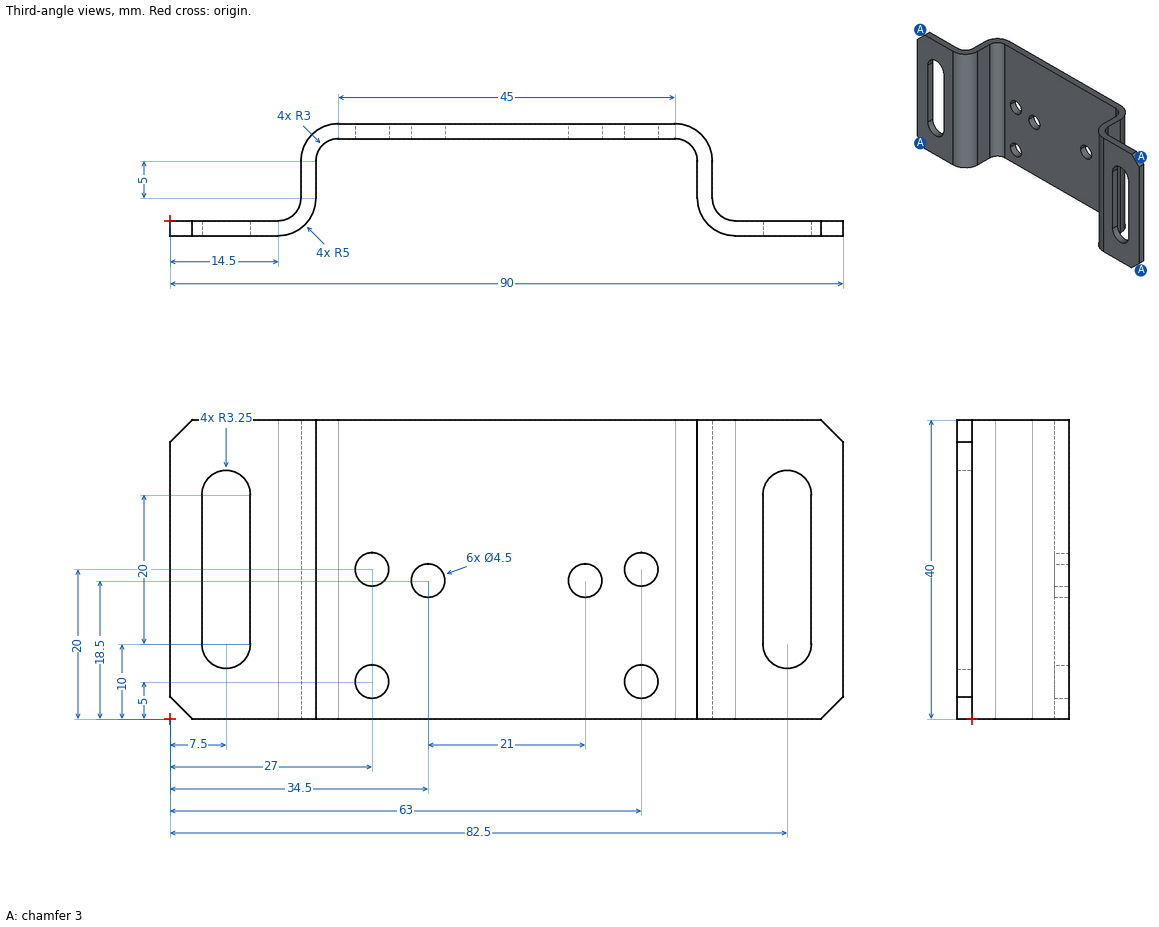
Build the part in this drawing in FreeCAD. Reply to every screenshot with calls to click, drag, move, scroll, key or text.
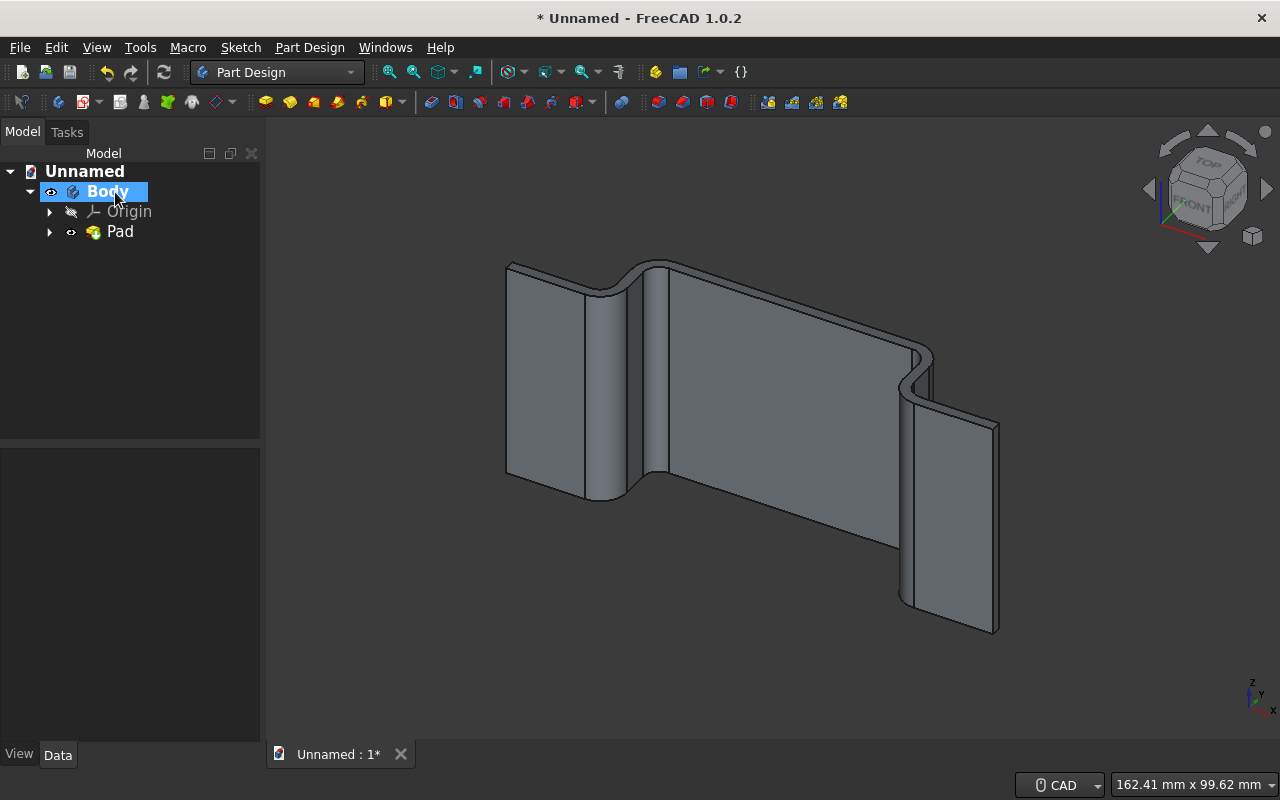
click(998, 424)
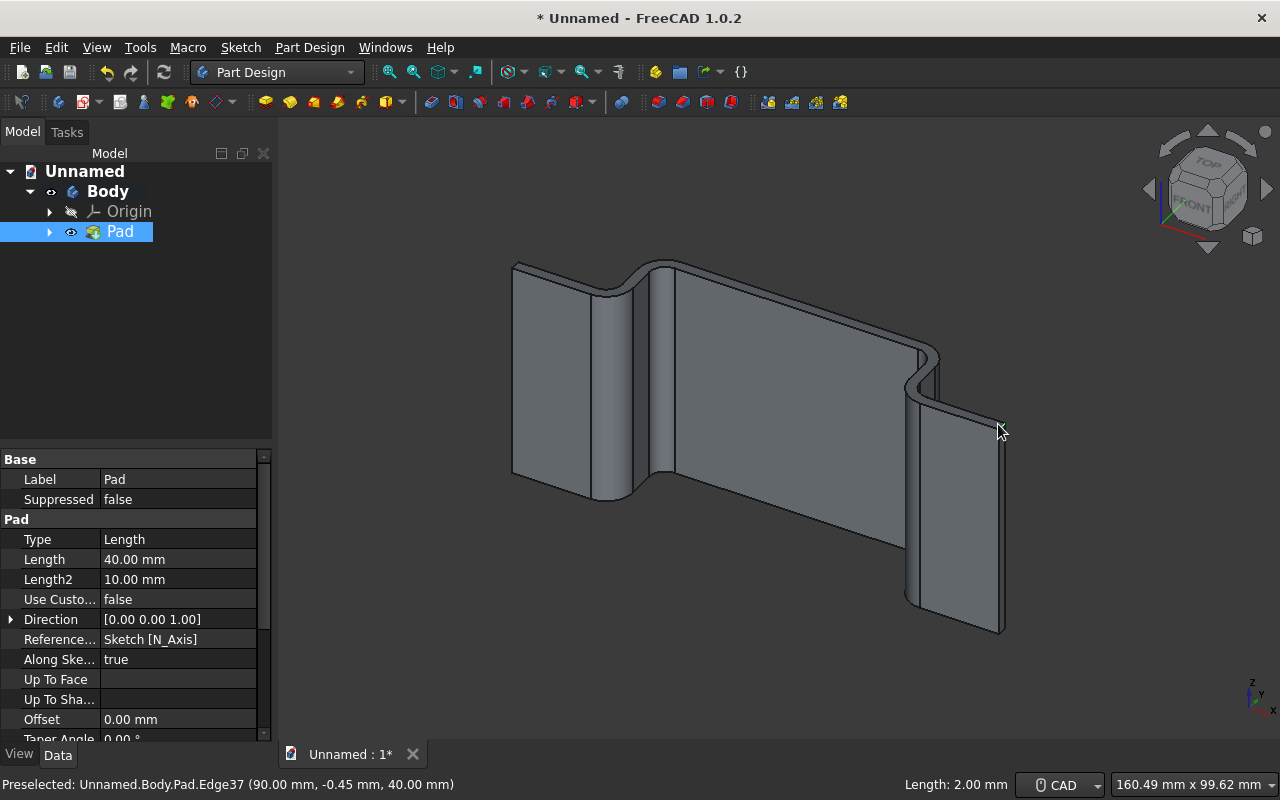
scroll(515, 469, up, 6)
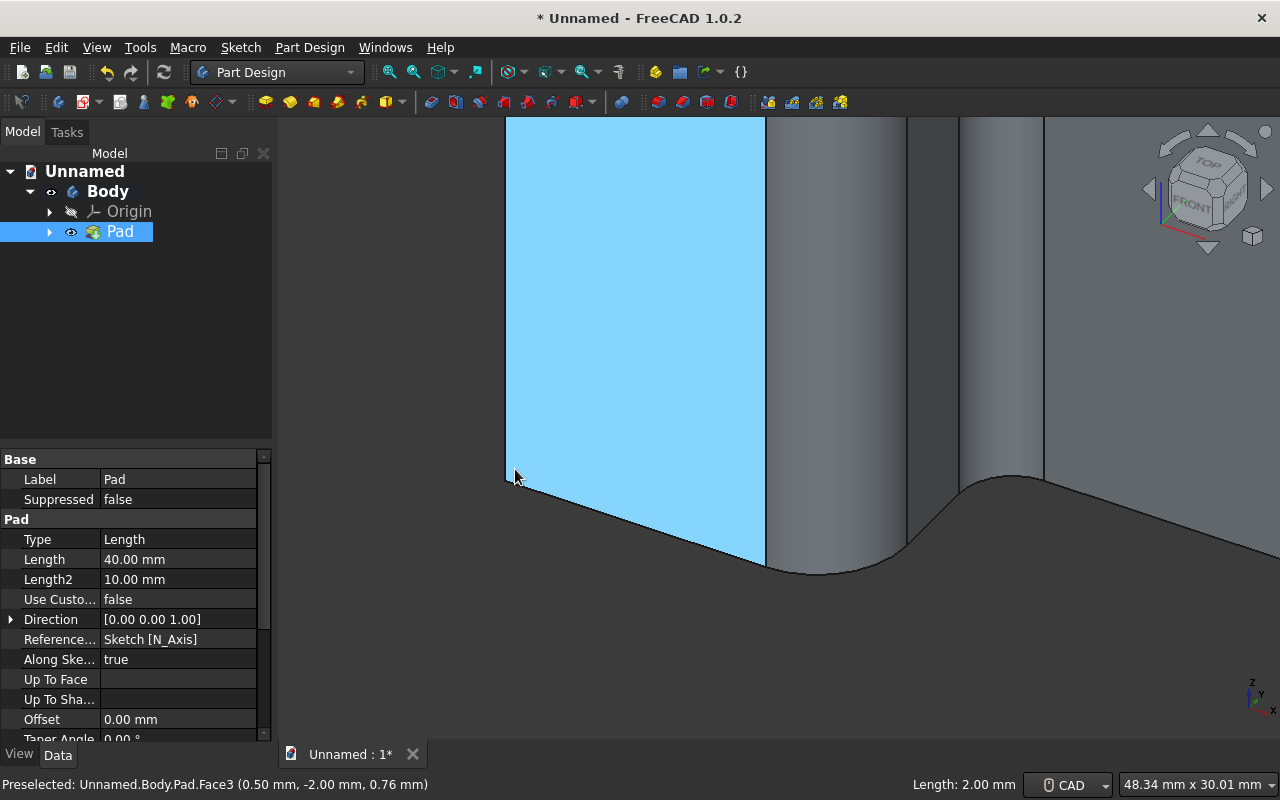
key(v)
key(f)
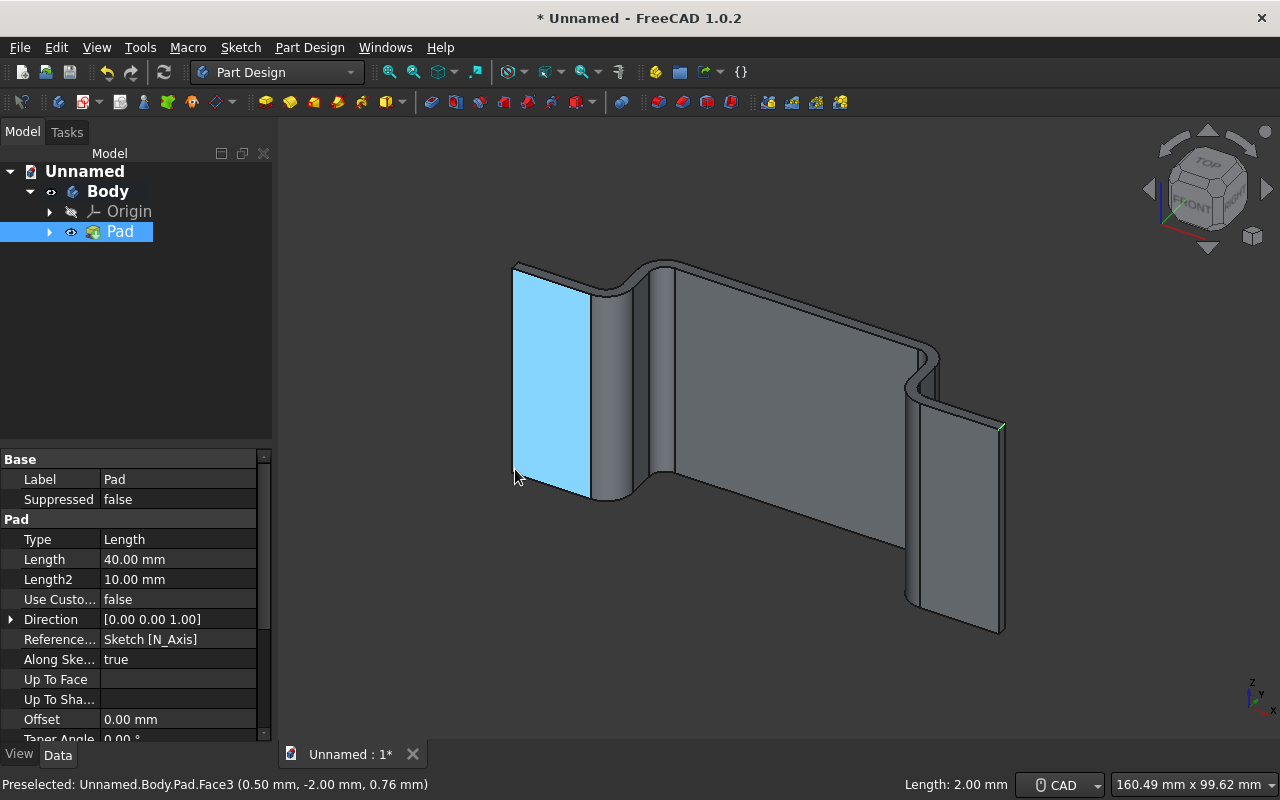
key(0)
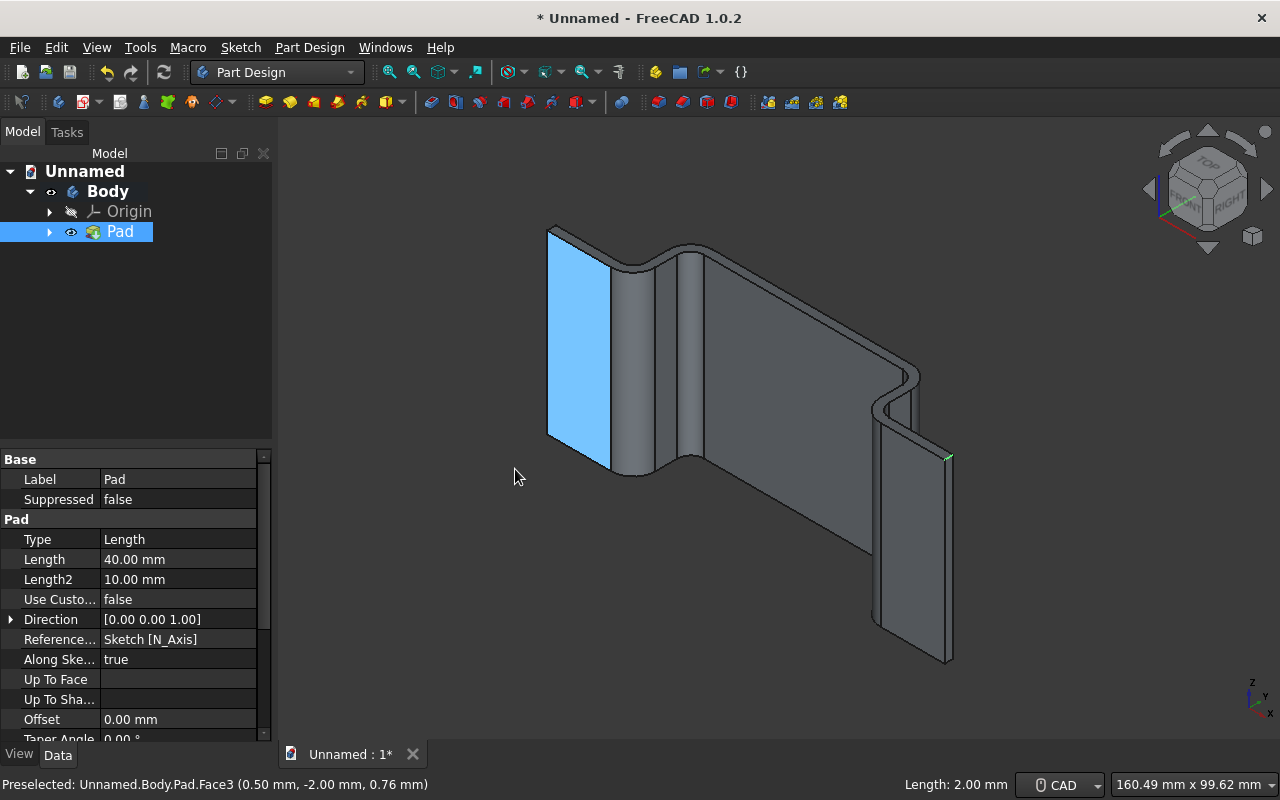
scroll(552, 431, up, 6)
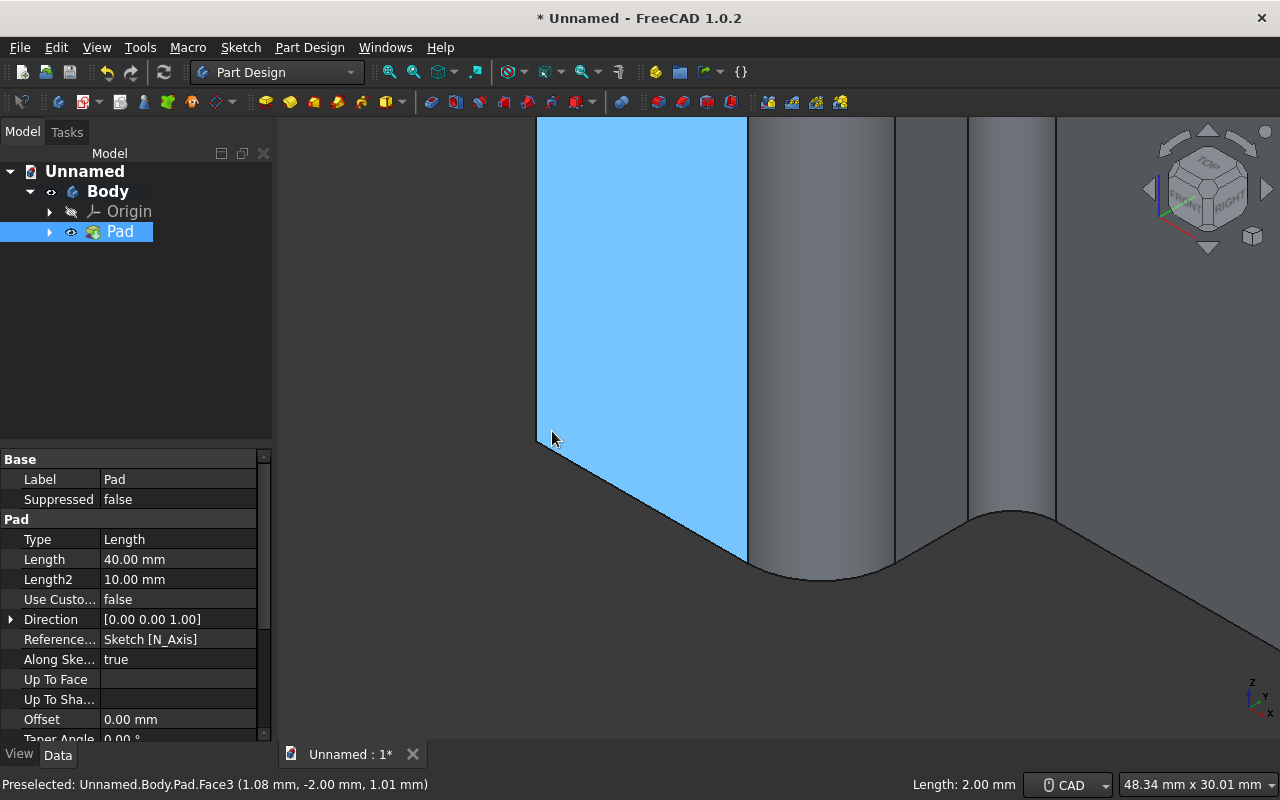
key(v)
key(f)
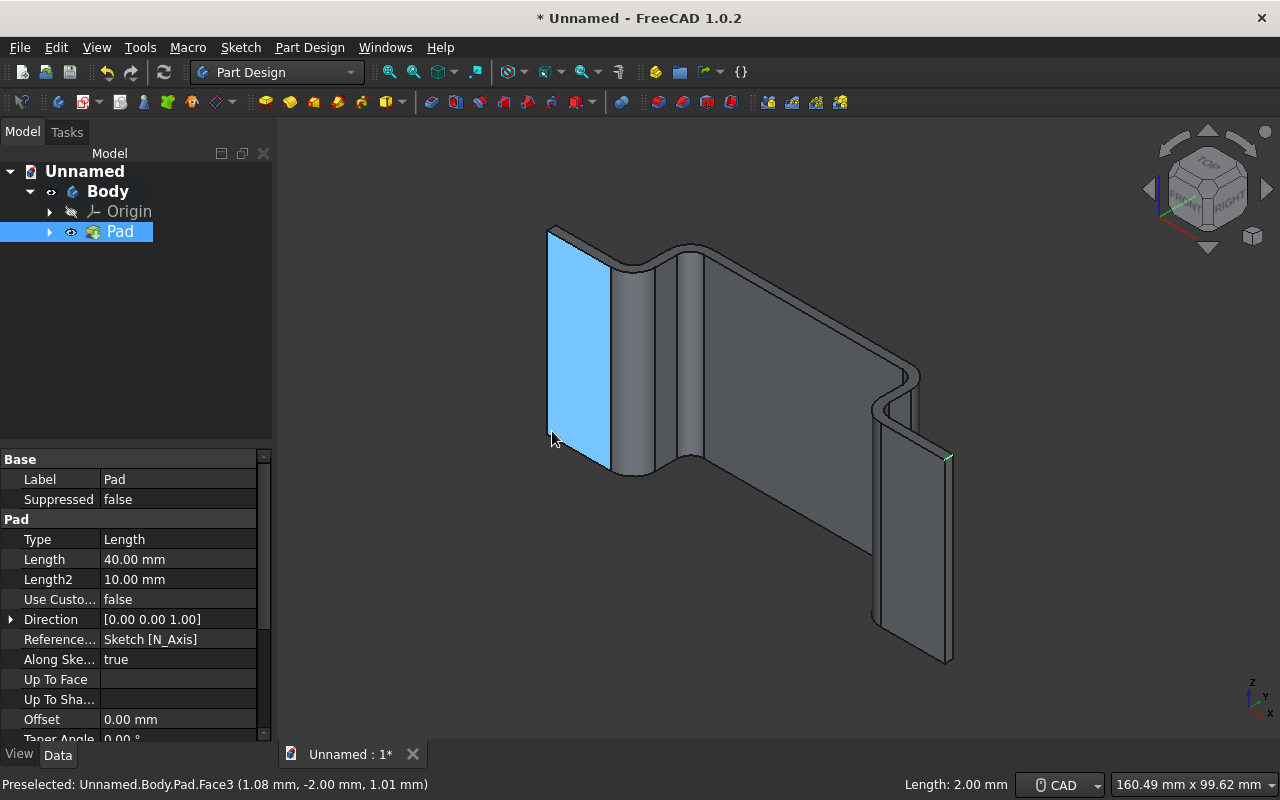
key(2)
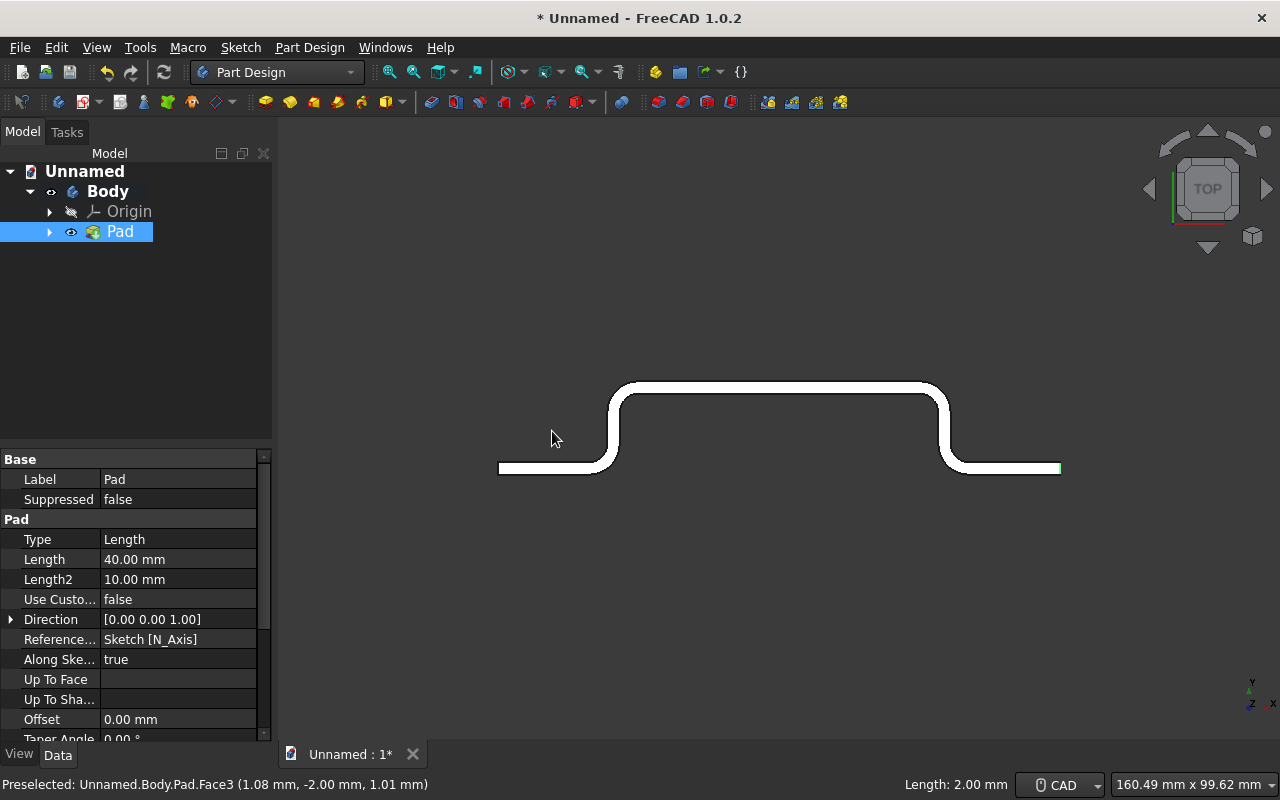
scroll(498, 468, up, 6)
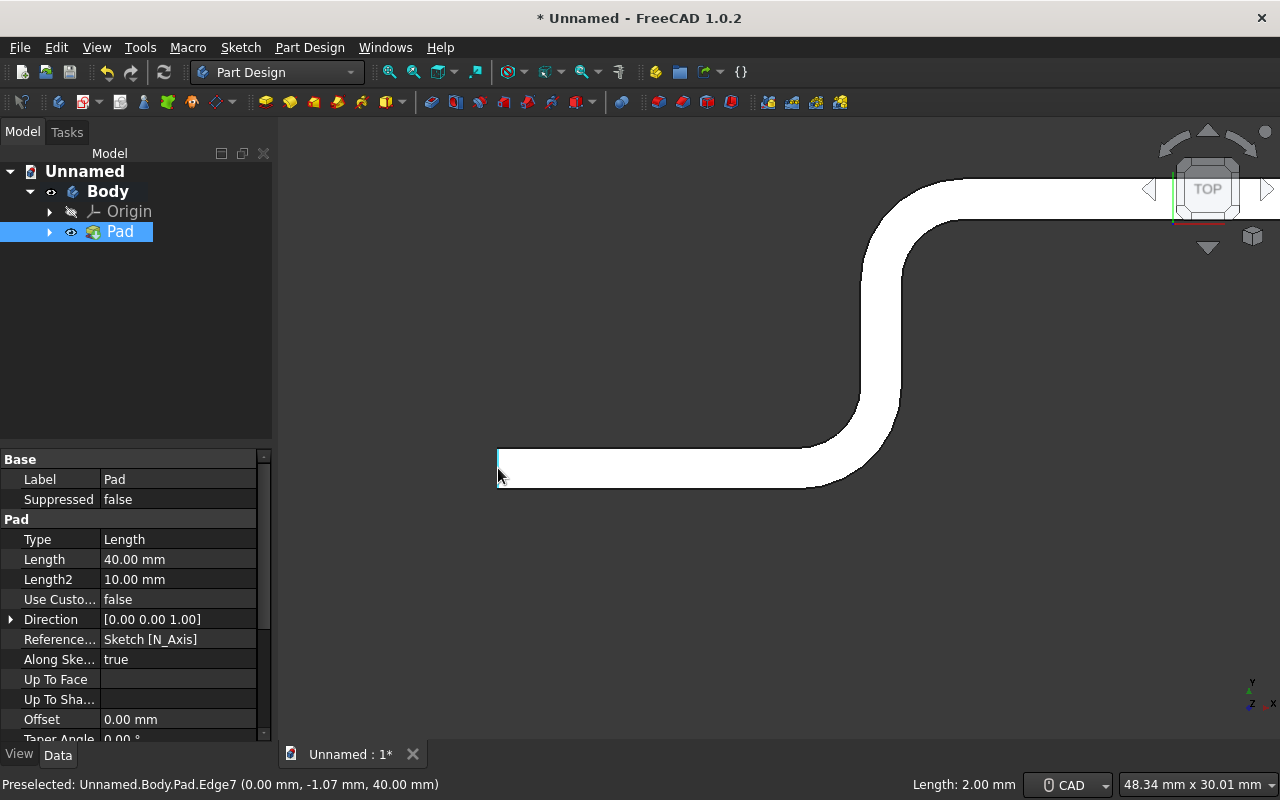
click(498, 468, ctrl)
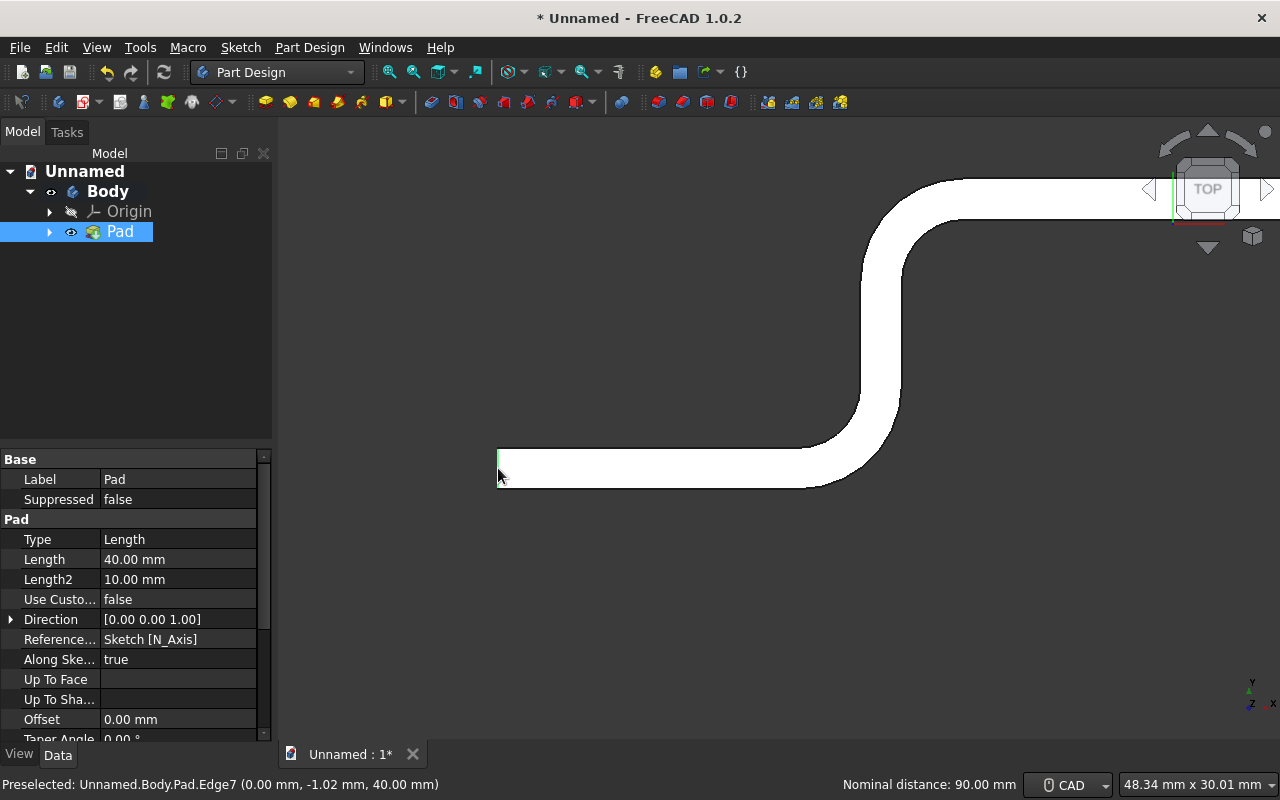
key(v)
key(f)